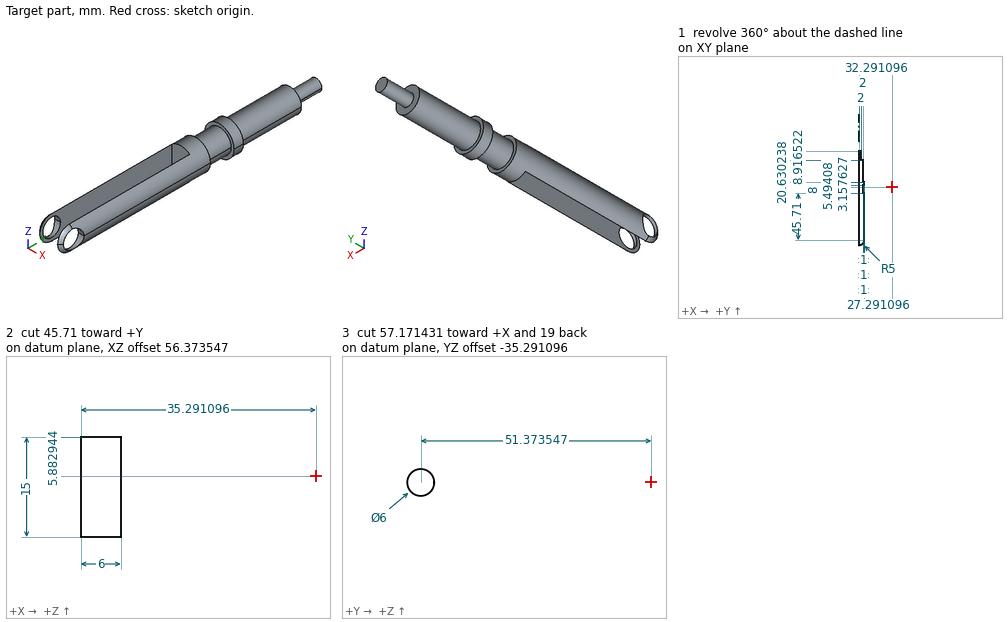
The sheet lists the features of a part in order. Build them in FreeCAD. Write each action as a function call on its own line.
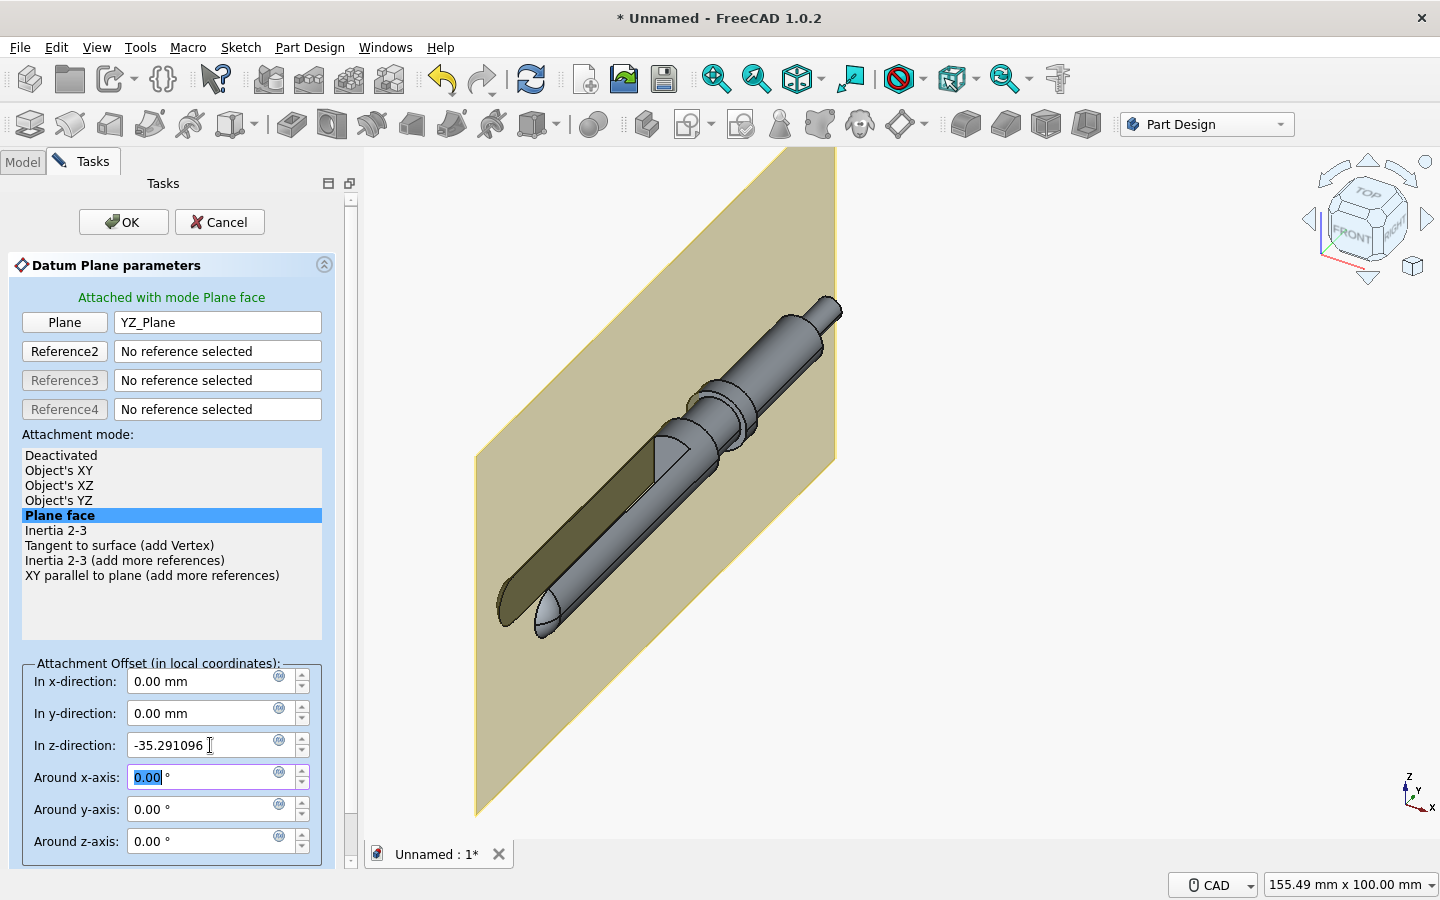
click(124, 222)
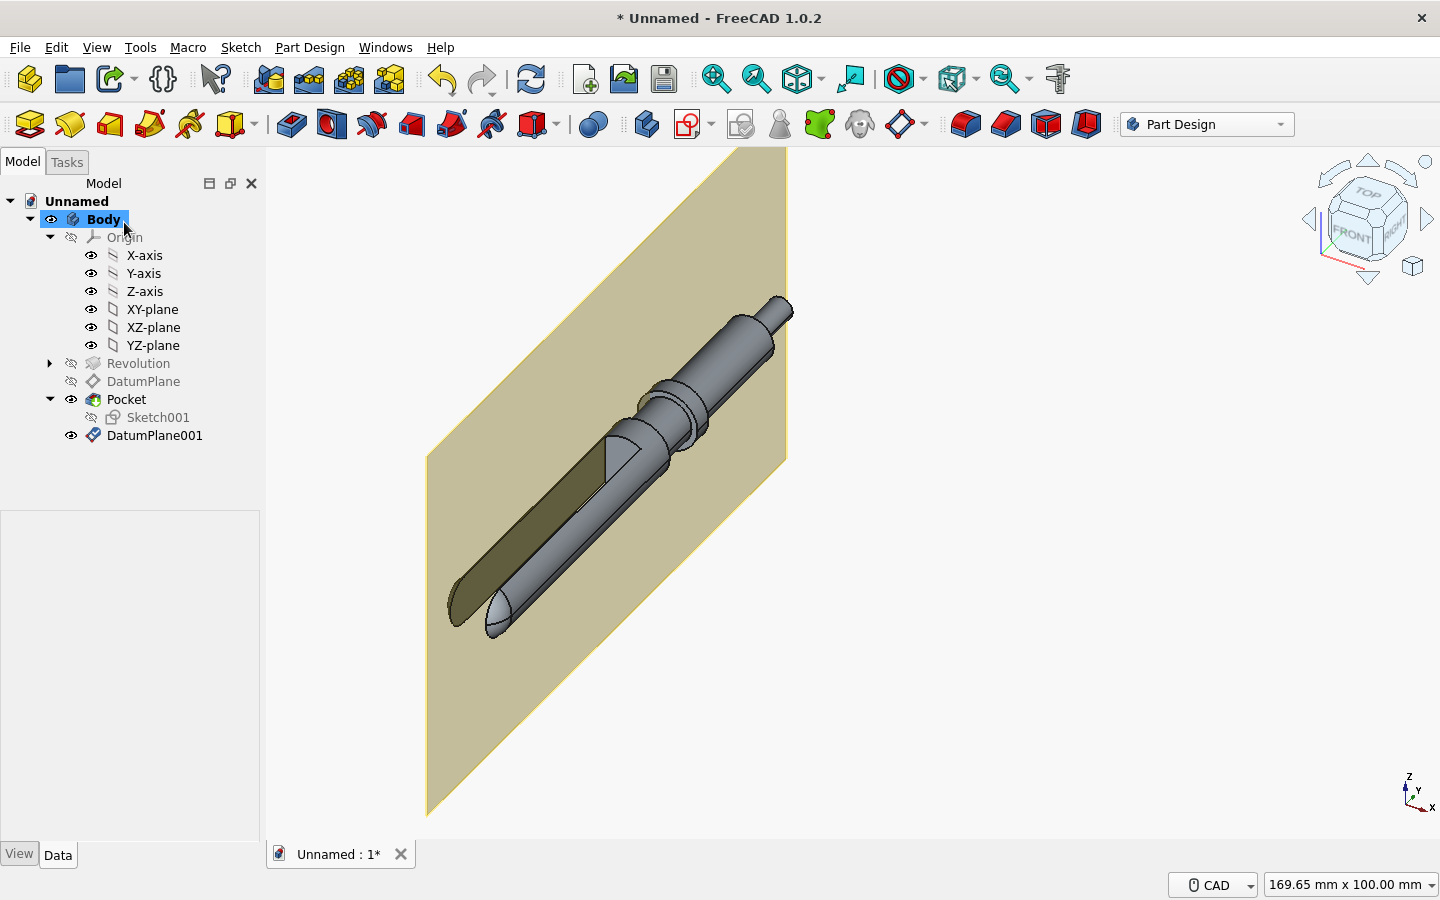
click(116, 435)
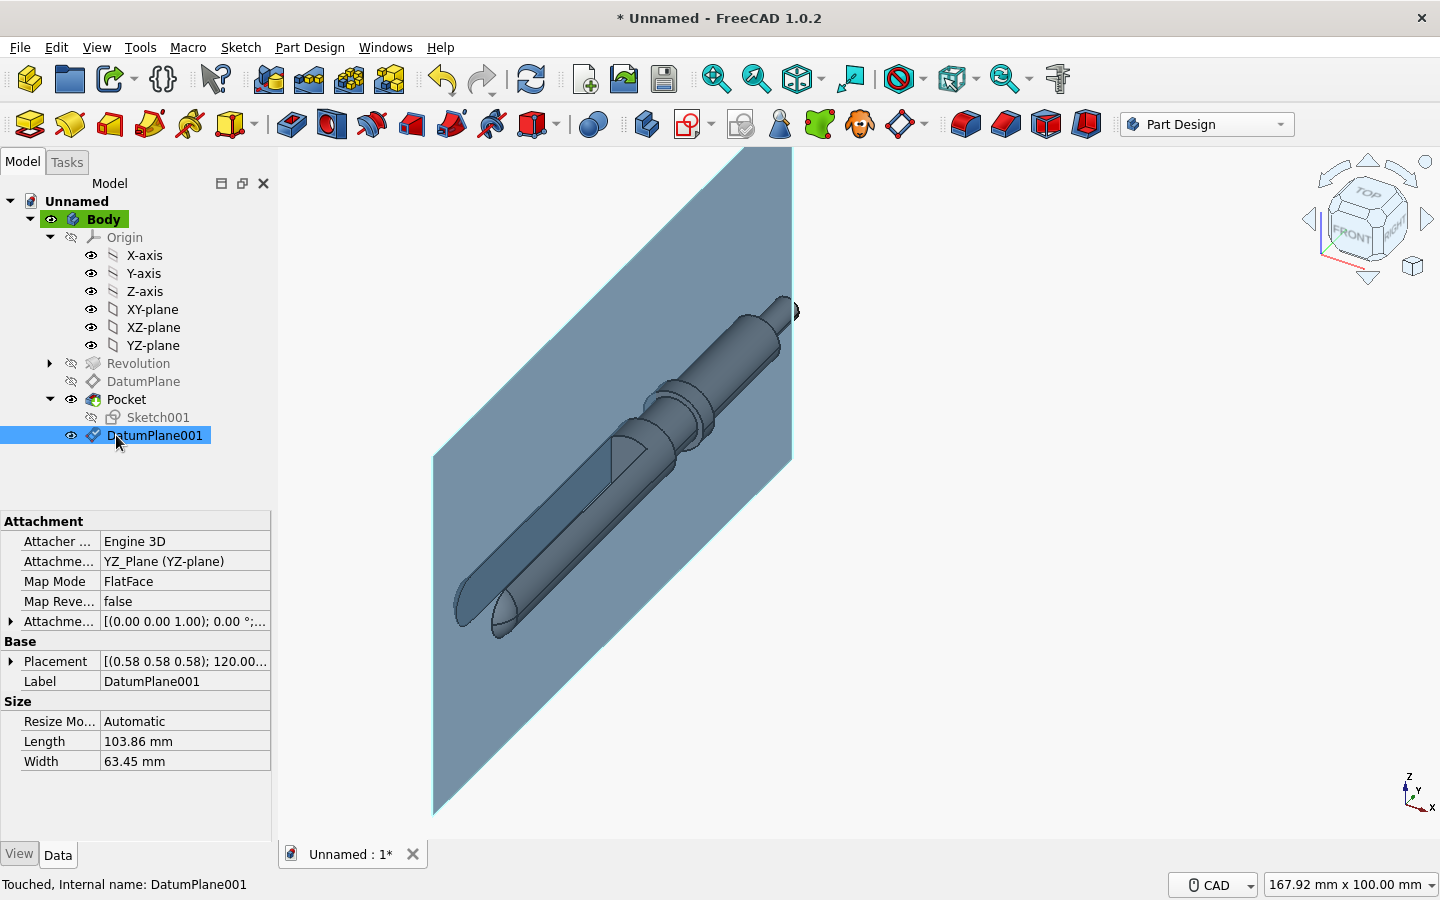
click(688, 124)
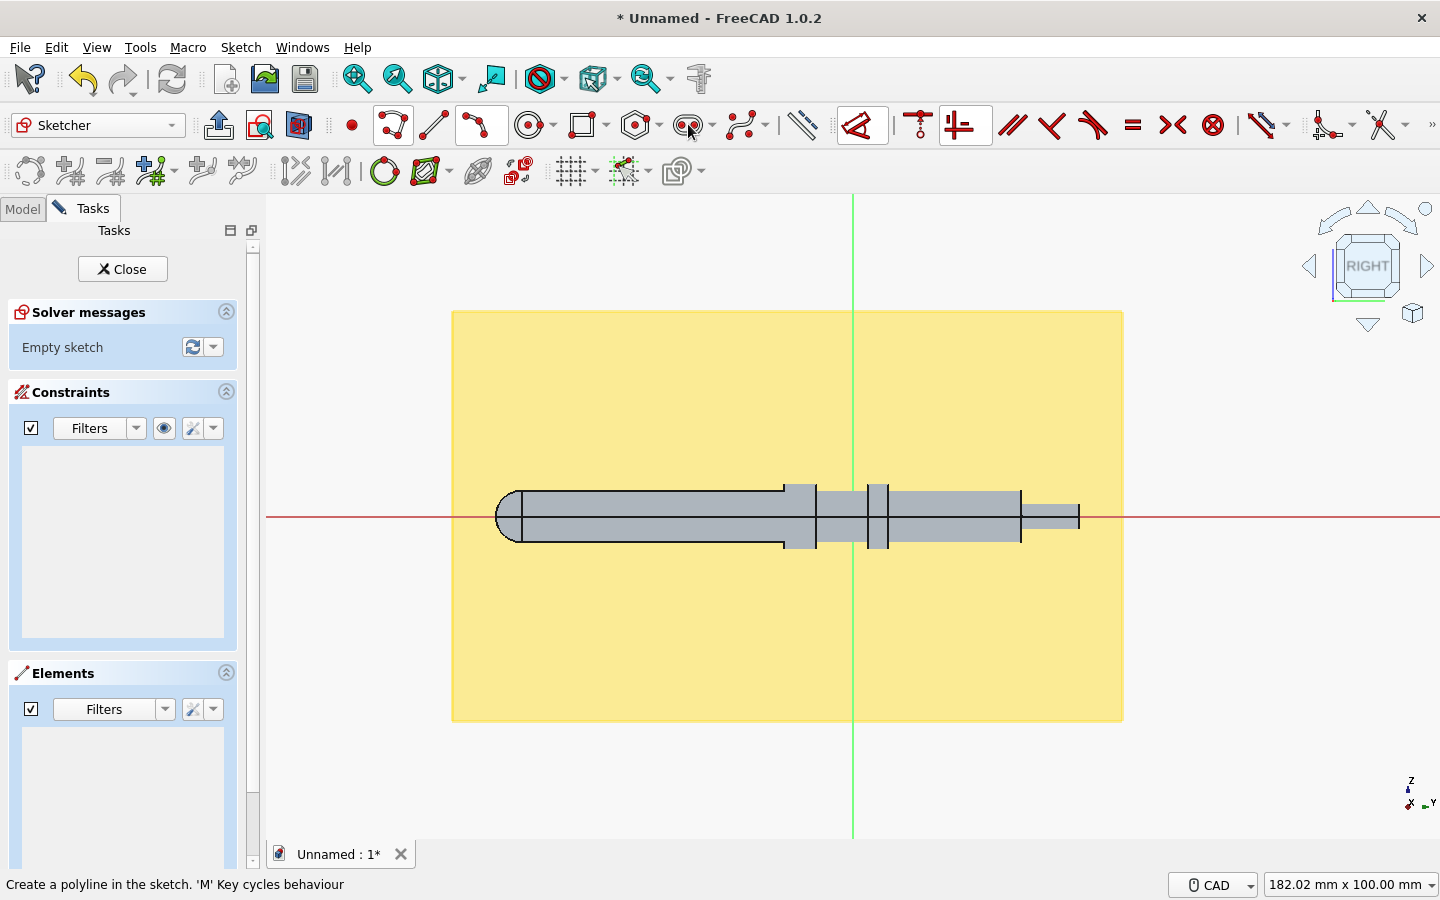
click(300, 126)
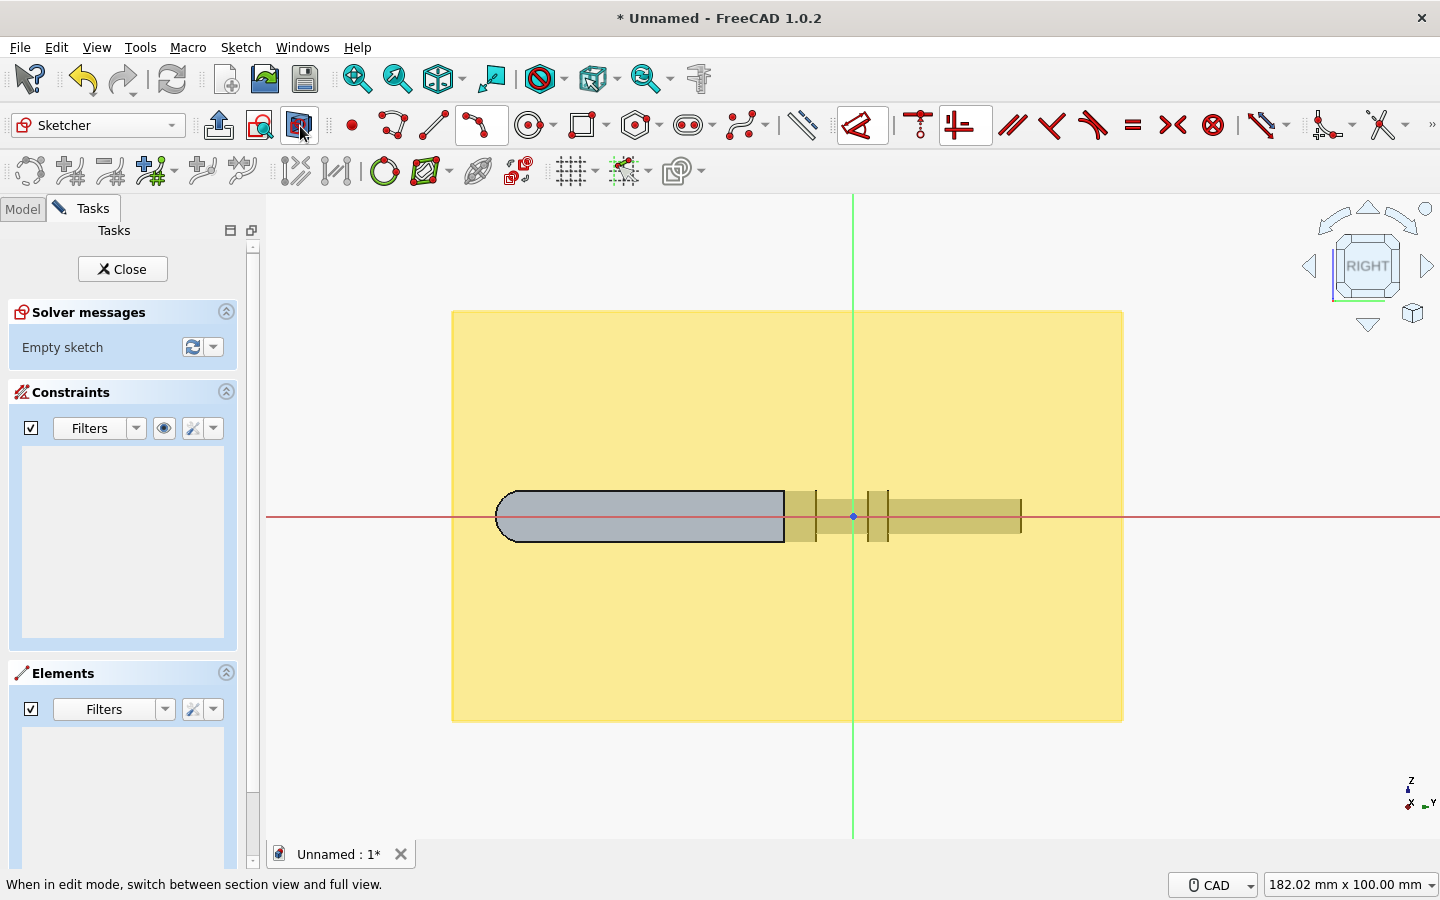
scroll(495, 516, up, 12)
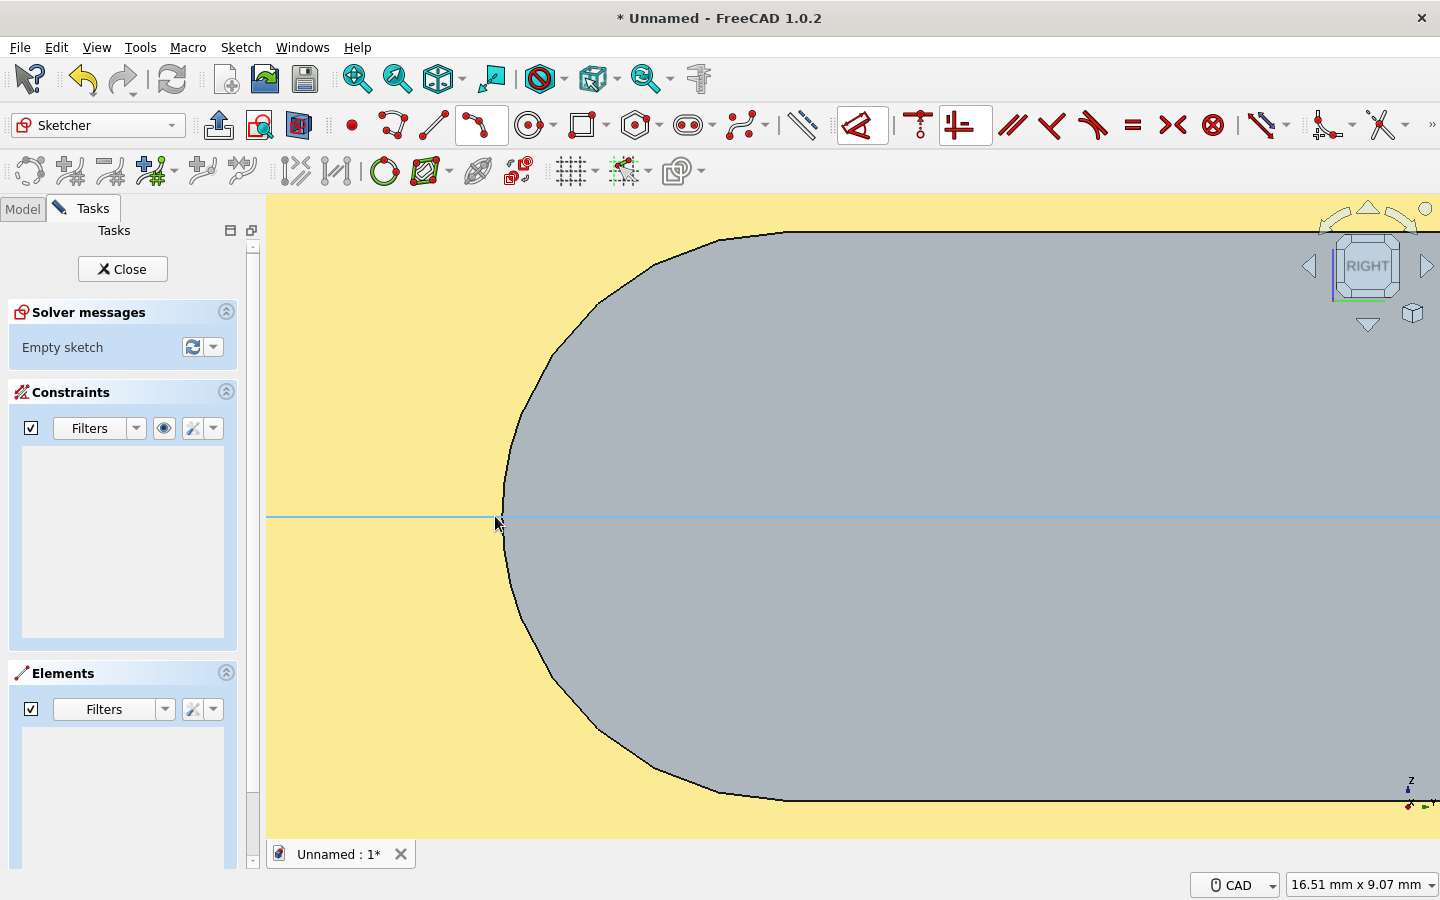
click(530, 126)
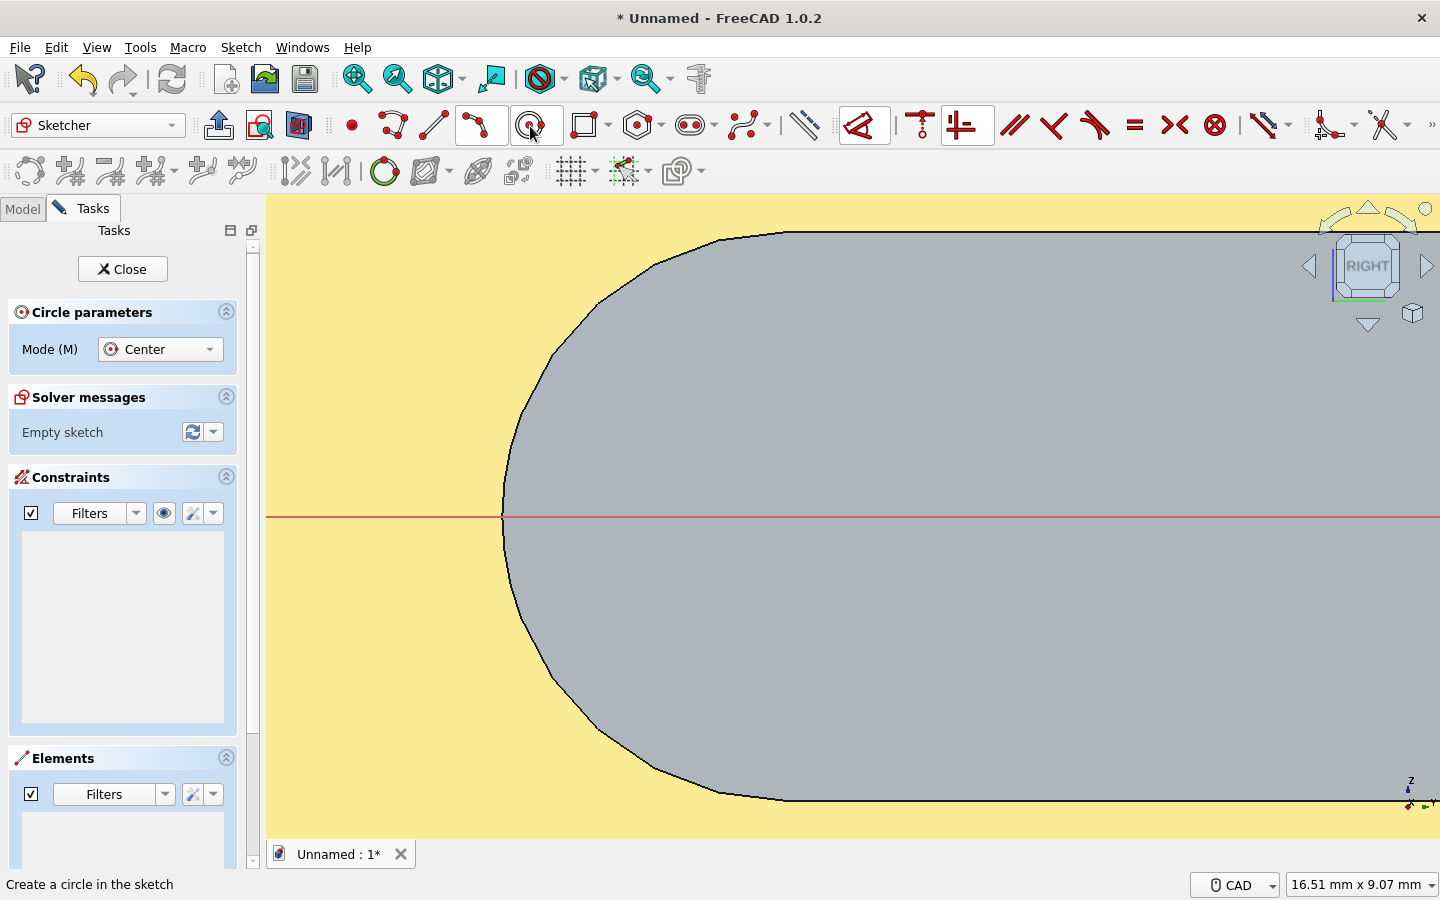
click(787, 516)
click(938, 366)
key(Escape)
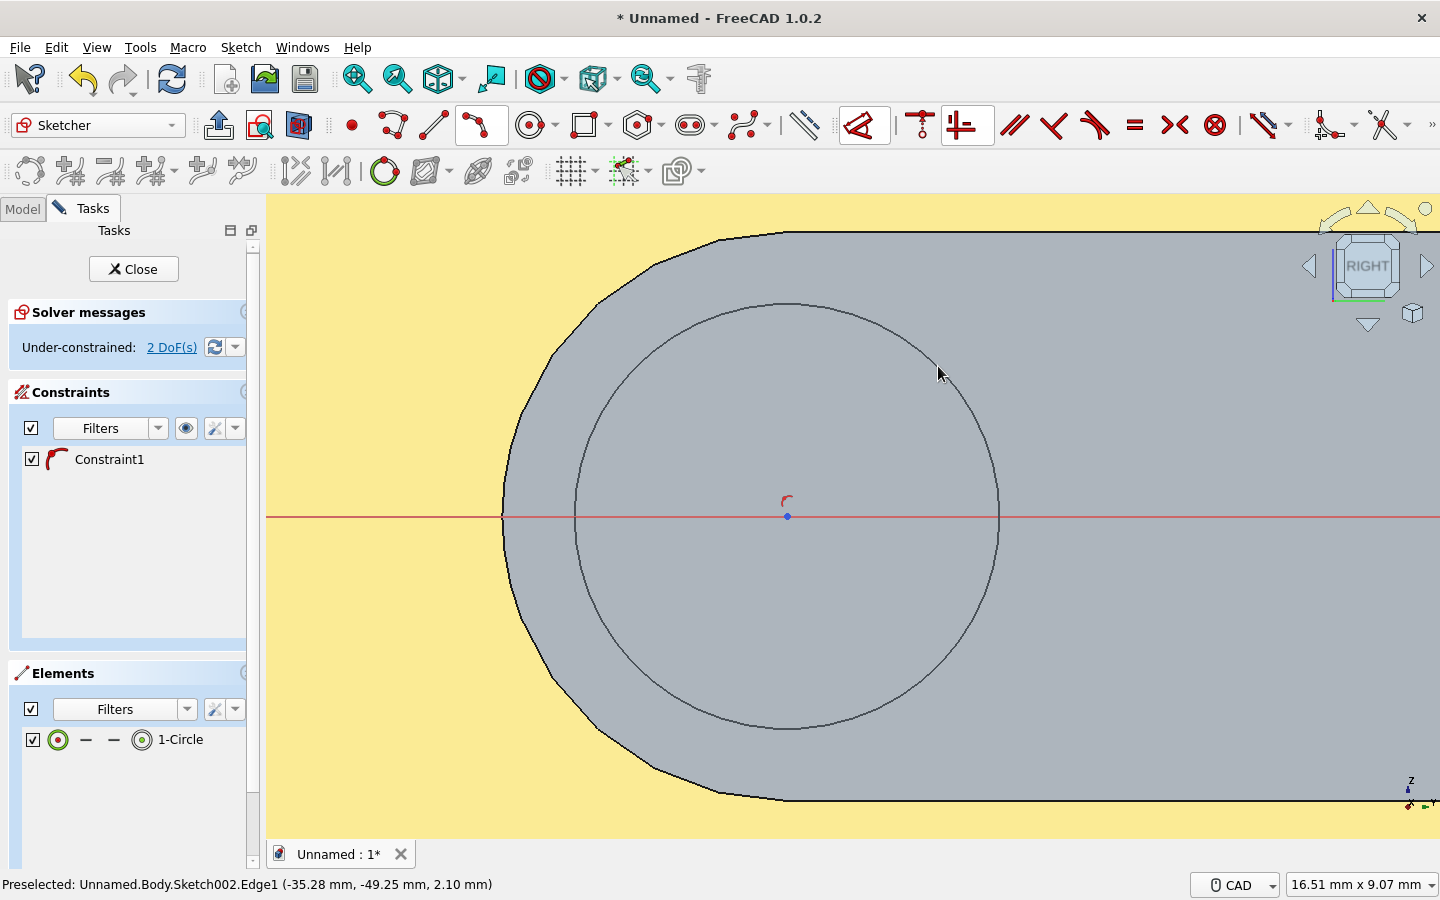
click(937, 366)